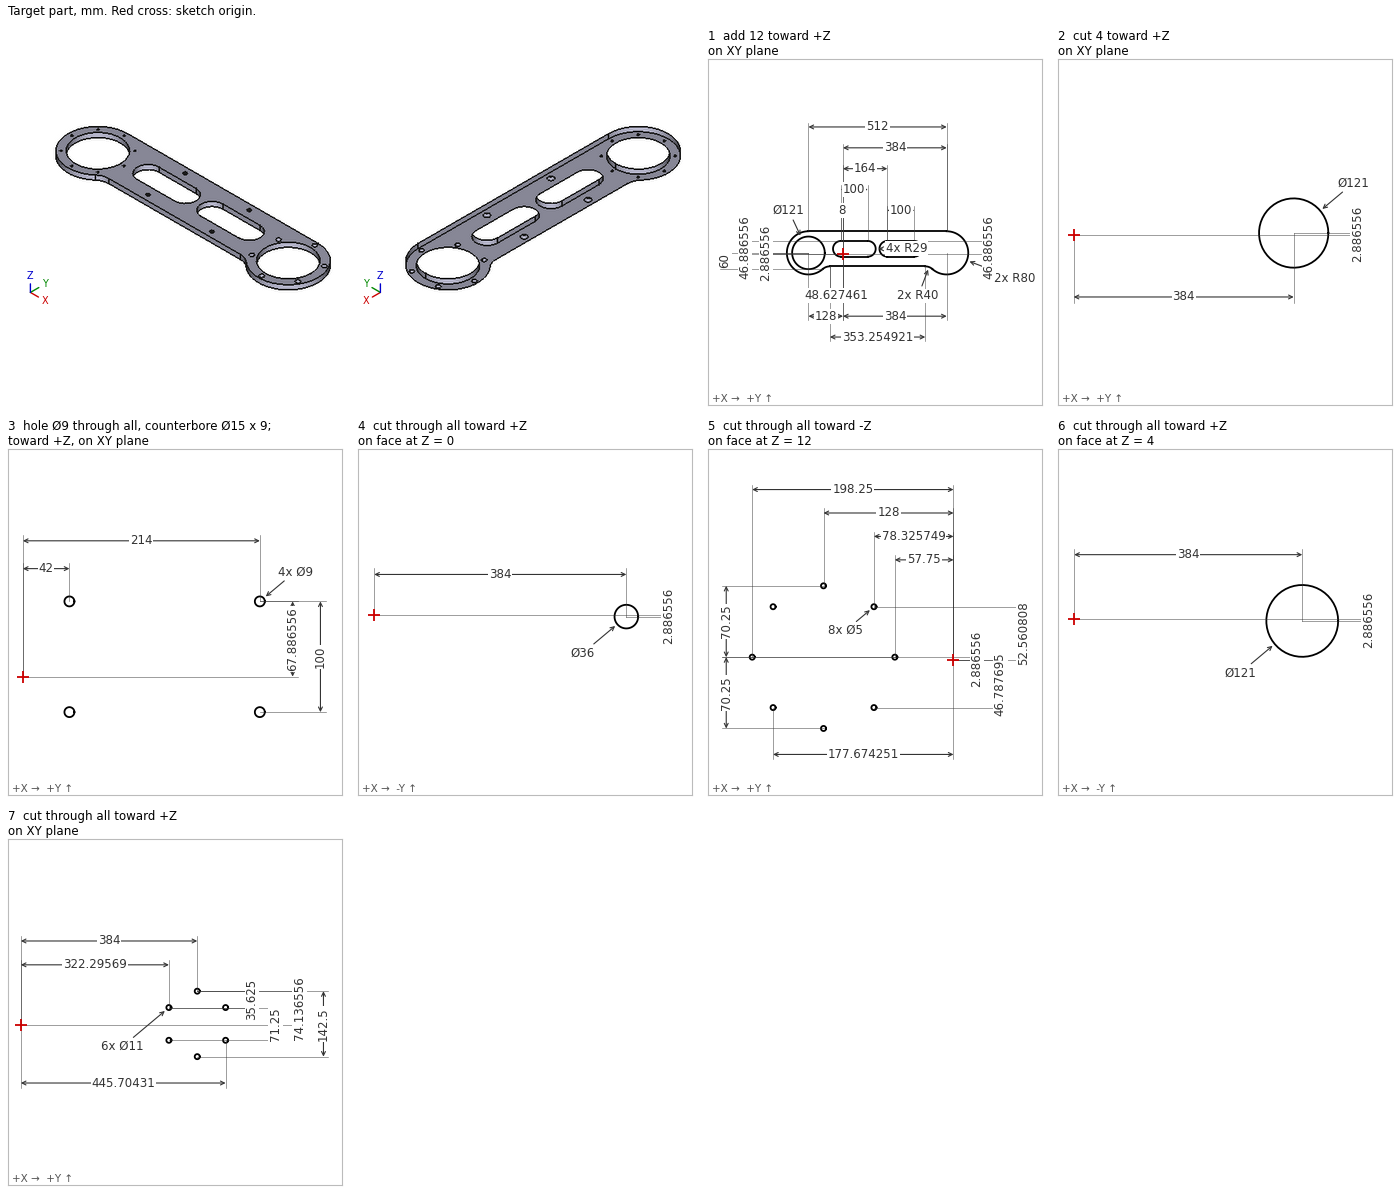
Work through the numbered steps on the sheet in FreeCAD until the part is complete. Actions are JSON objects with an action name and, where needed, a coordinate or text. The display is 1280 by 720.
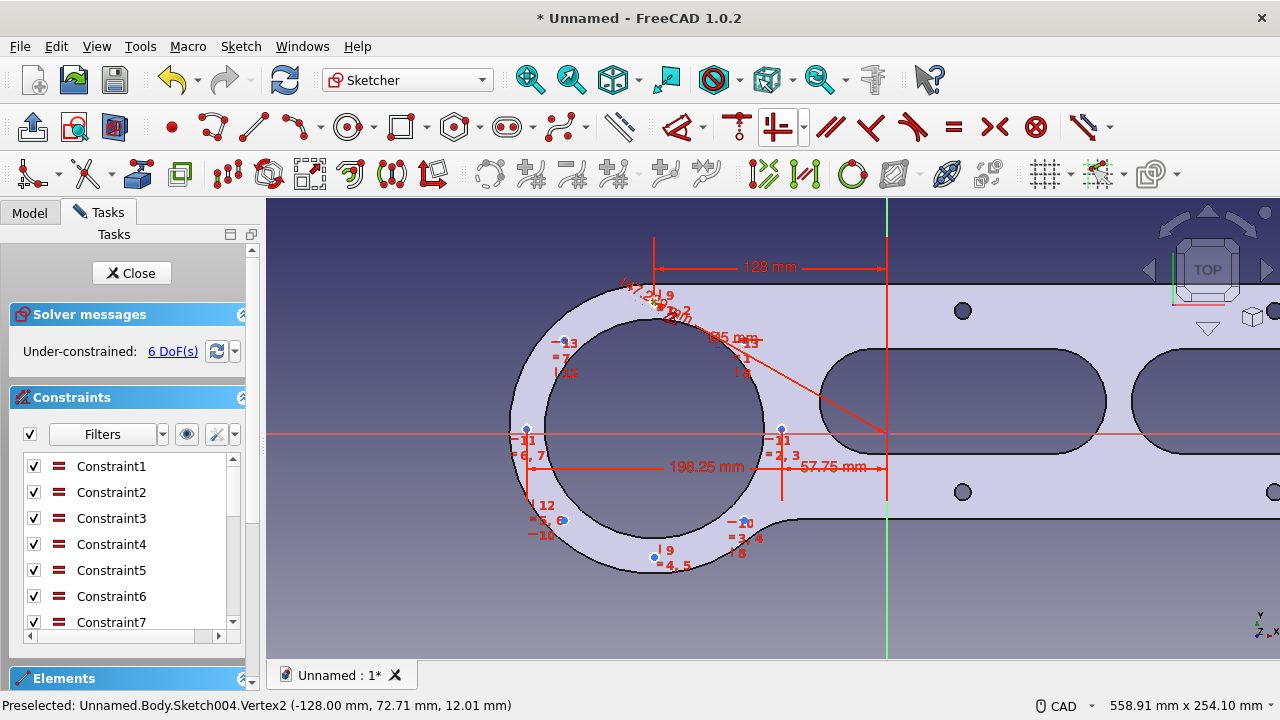
{"action": "left_click", "coordinate": [782, 429]}
{"action": "left_click", "coordinate": [816, 366]}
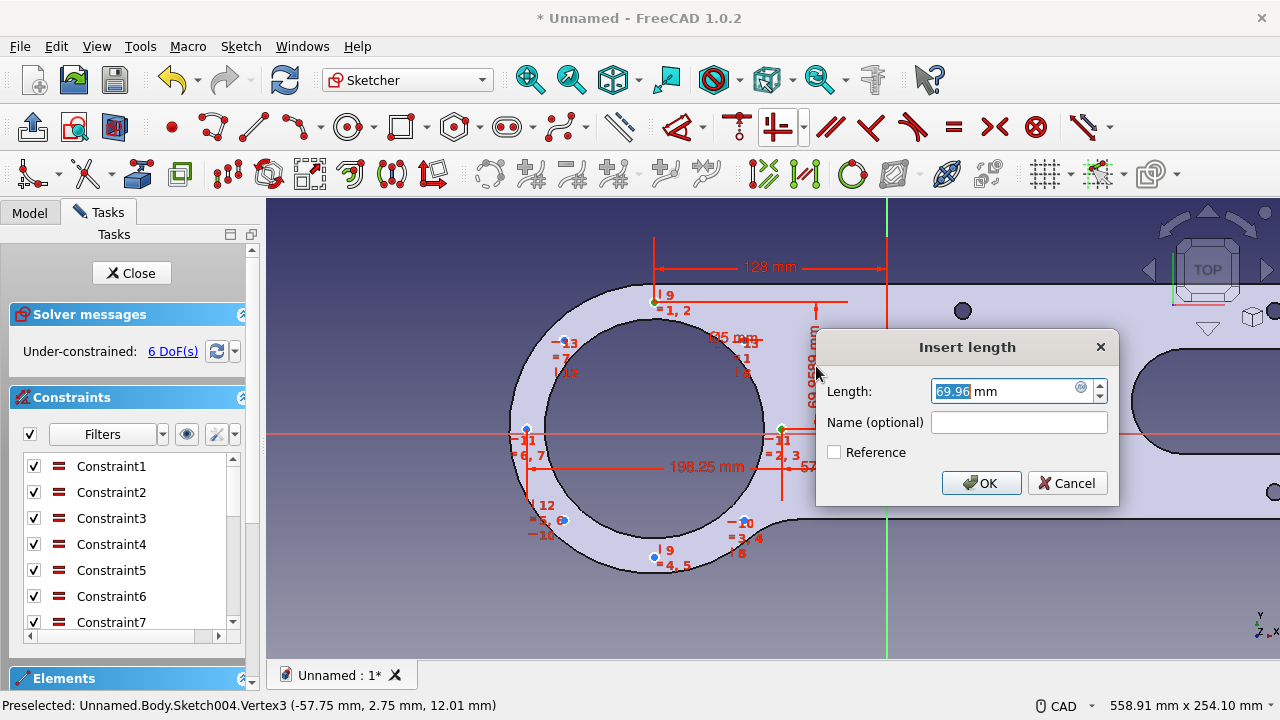
{"action": "type", "text": "70.25"}
{"action": "key", "text": "Return"}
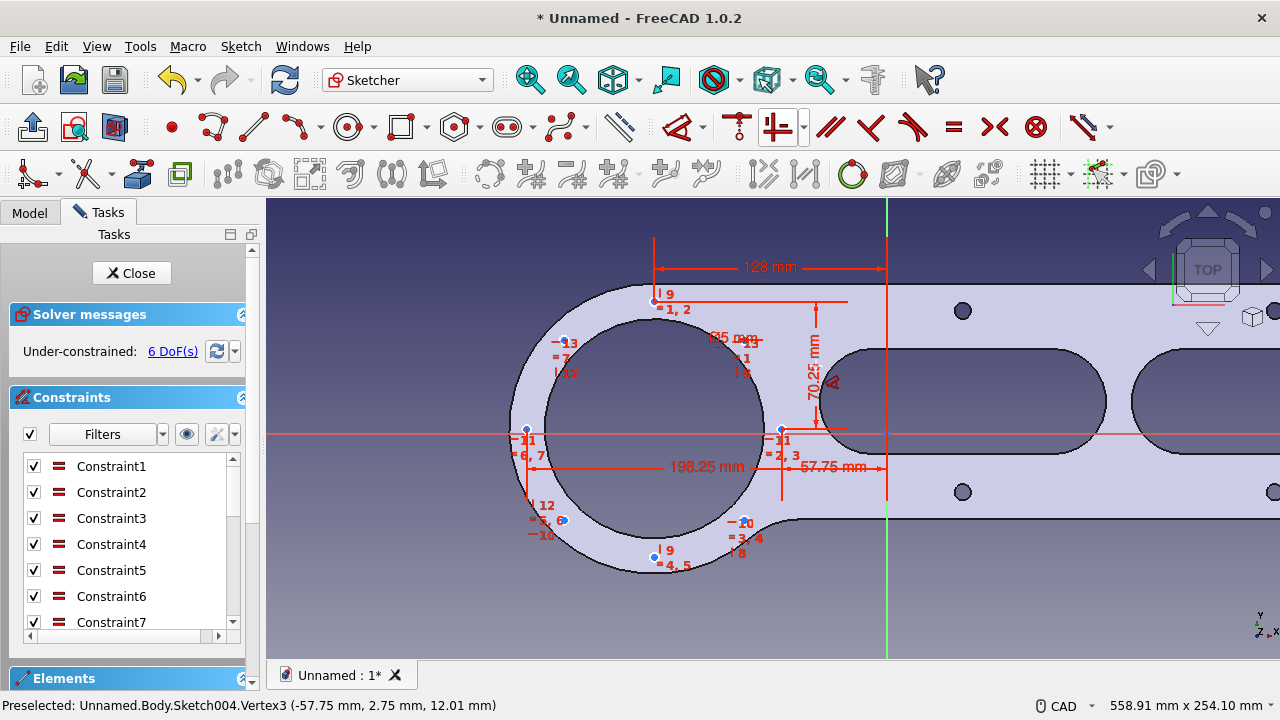
{"action": "left_click", "coordinate": [782, 429]}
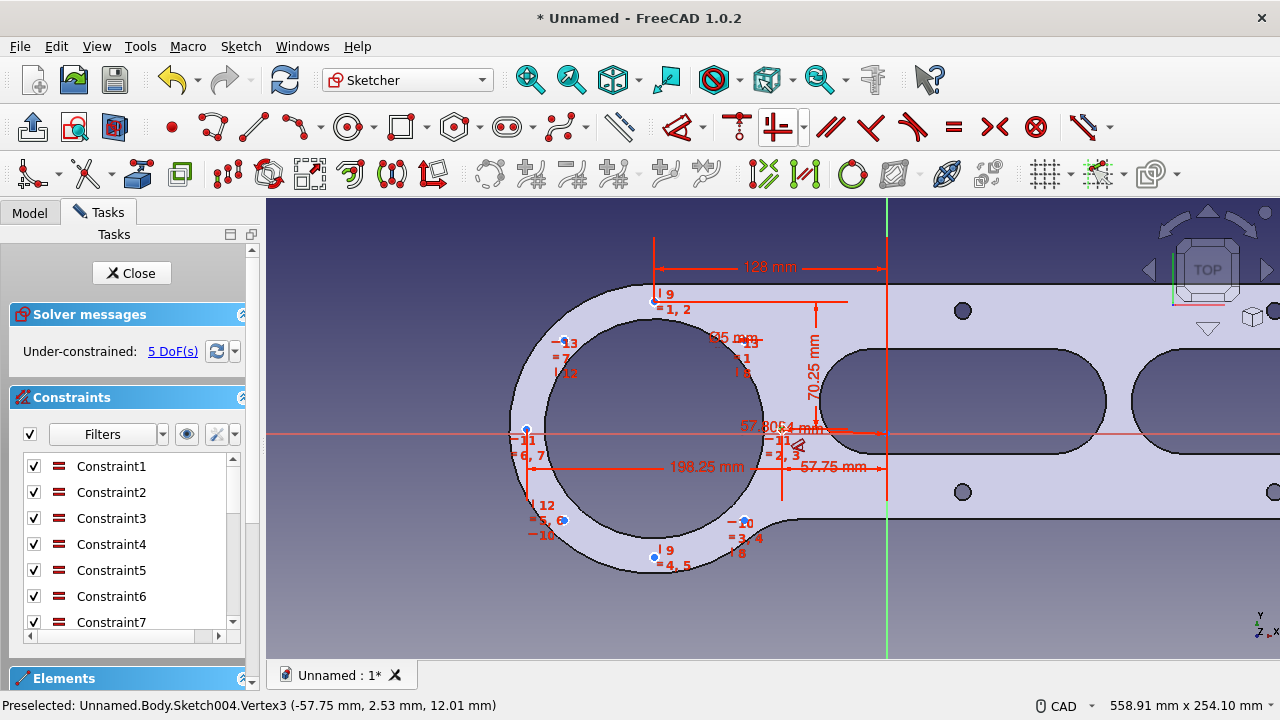
{"action": "left_click", "coordinate": [654, 557]}
{"action": "left_click", "coordinate": [816, 493]}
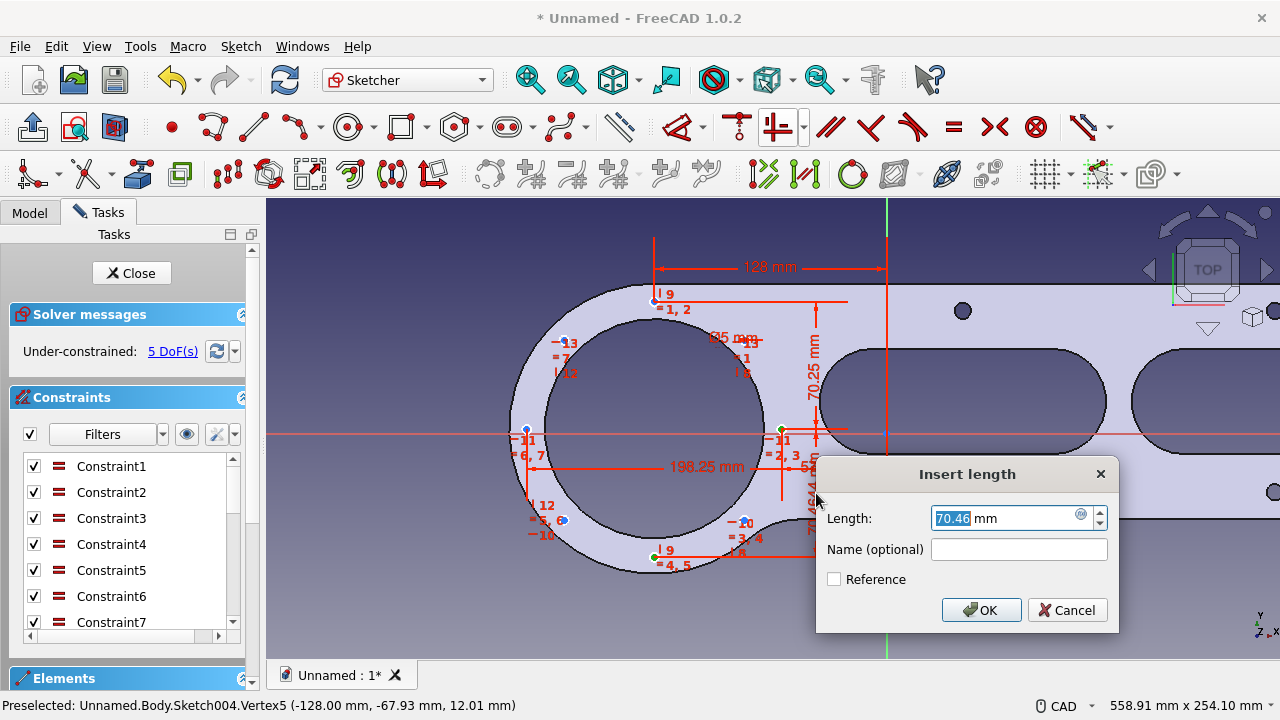
{"action": "type", "text": "70.25"}
{"action": "key", "text": "Return"}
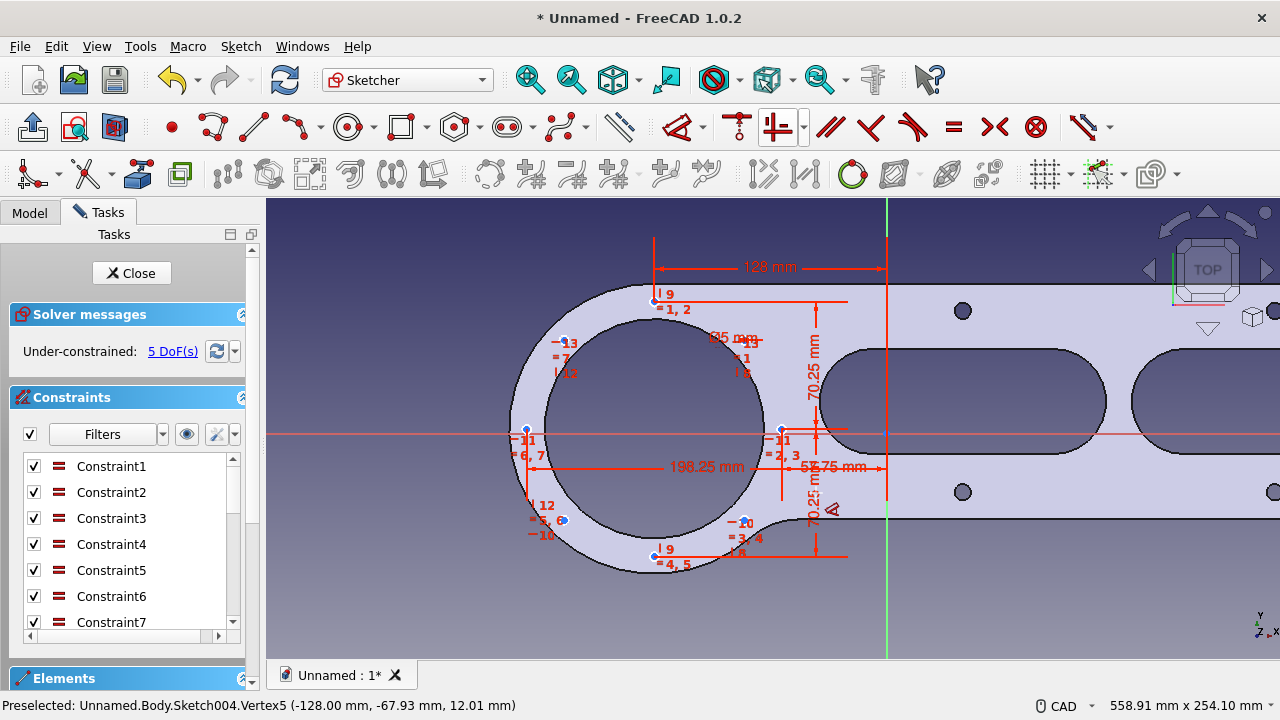
{"action": "scroll", "coordinate": [782, 429], "scroll_direction": "up", "scroll_amount": 11}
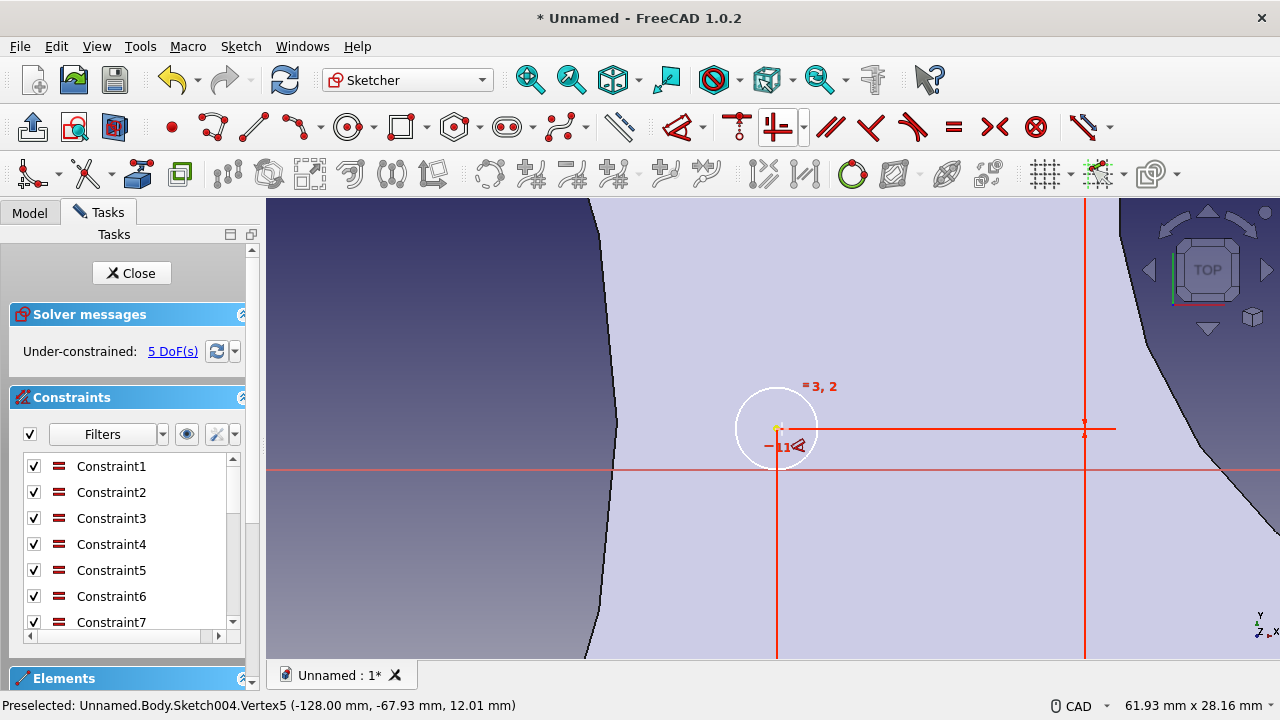
{"action": "left_click", "coordinate": [777, 429]}
{"action": "left_click", "coordinate": [719, 449]}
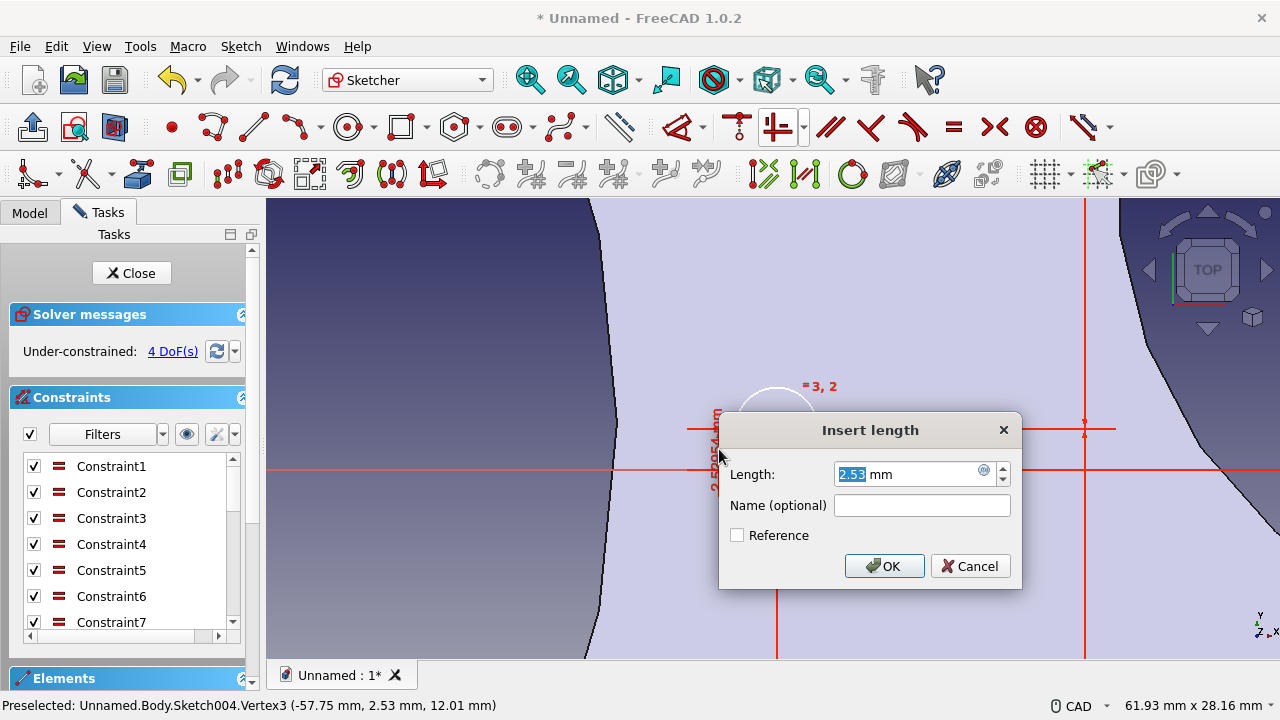
{"action": "type", "text": "2.886556"}
{"action": "key", "text": "Return"}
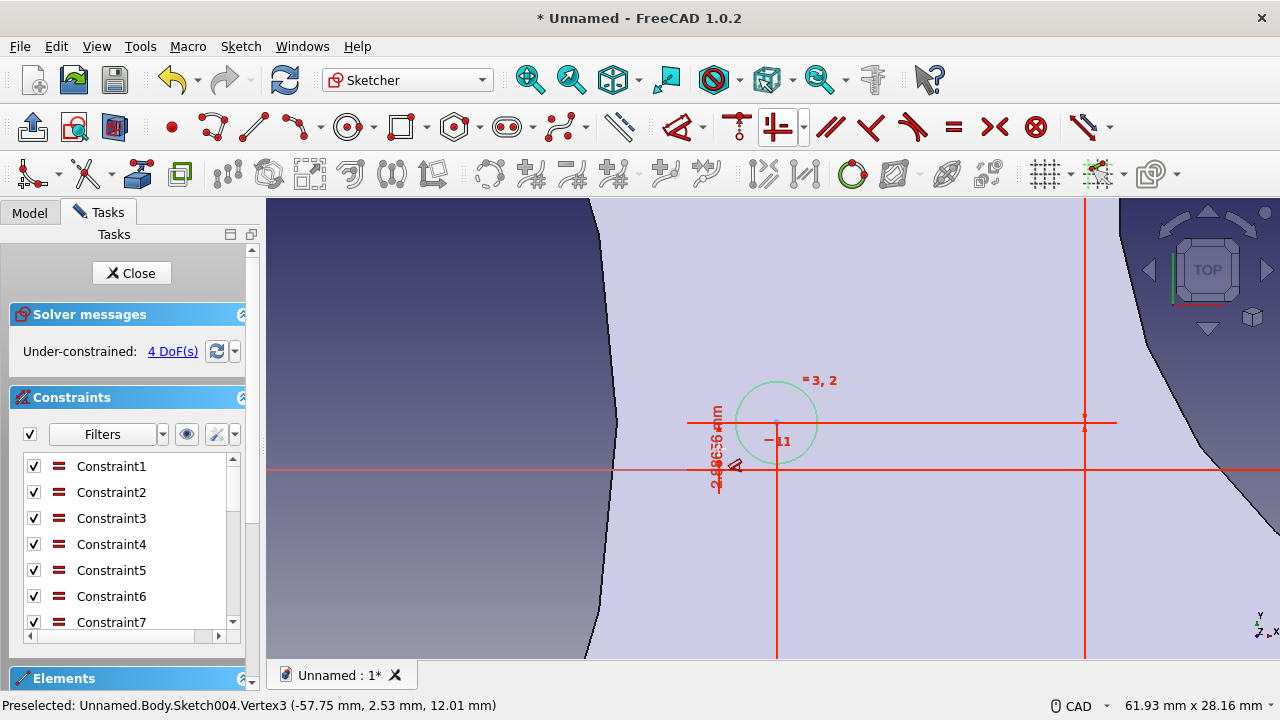
{"action": "scroll", "coordinate": [782, 429], "scroll_direction": "down", "scroll_amount": 11}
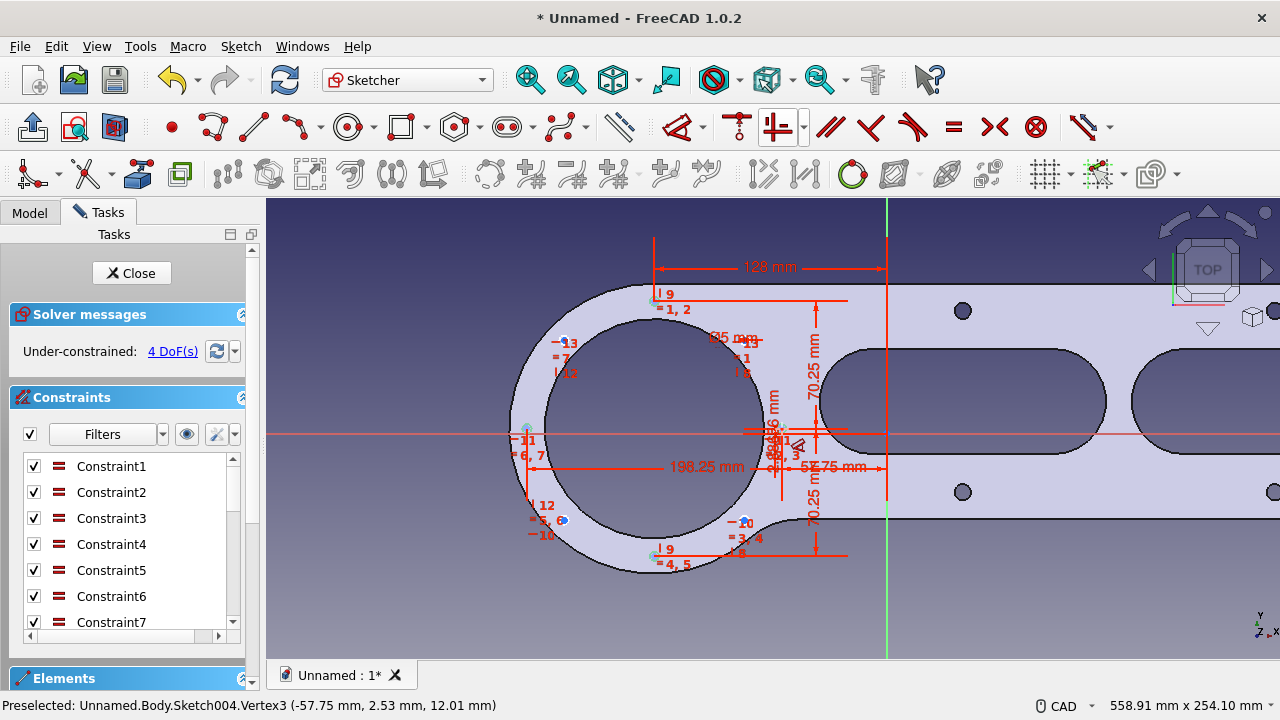
{"action": "left_click", "coordinate": [744, 340]}
{"action": "left_click", "coordinate": [815, 306]}